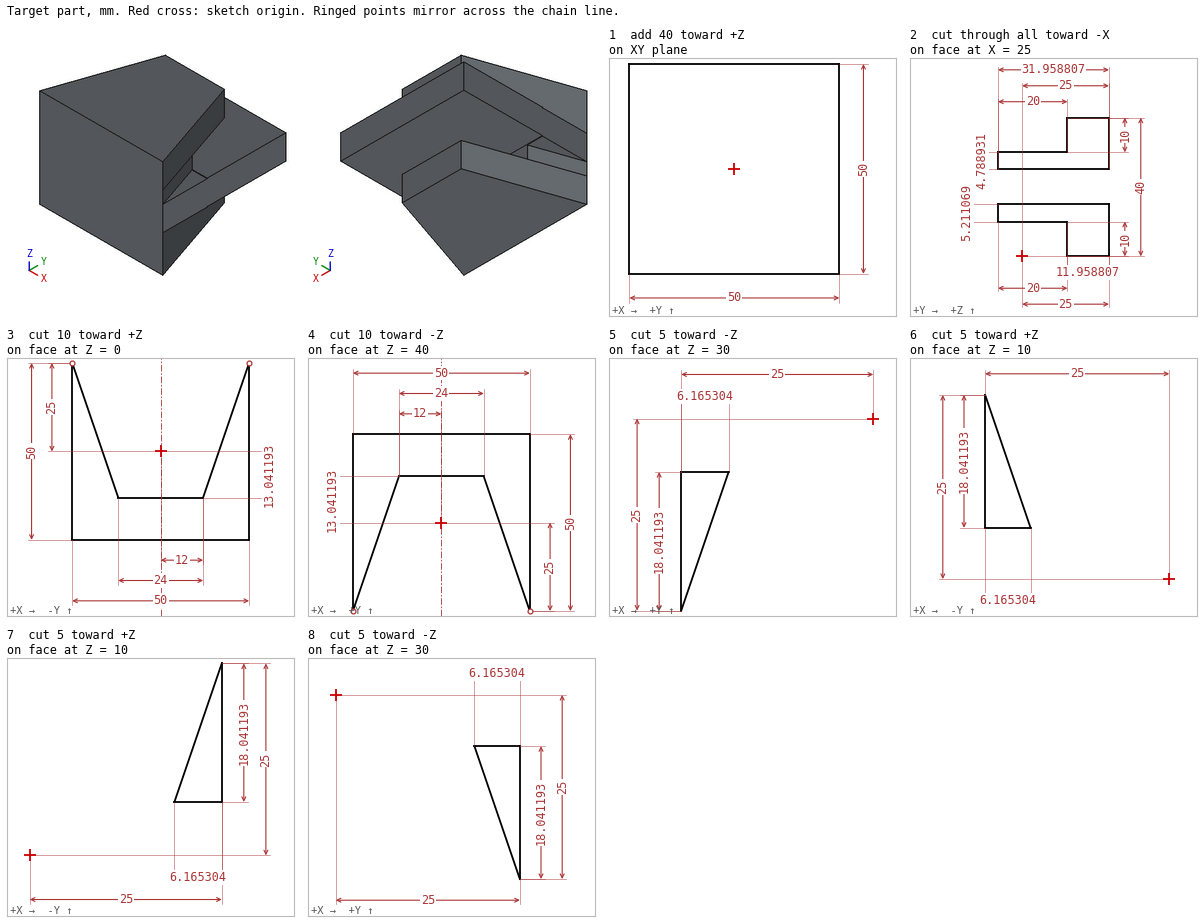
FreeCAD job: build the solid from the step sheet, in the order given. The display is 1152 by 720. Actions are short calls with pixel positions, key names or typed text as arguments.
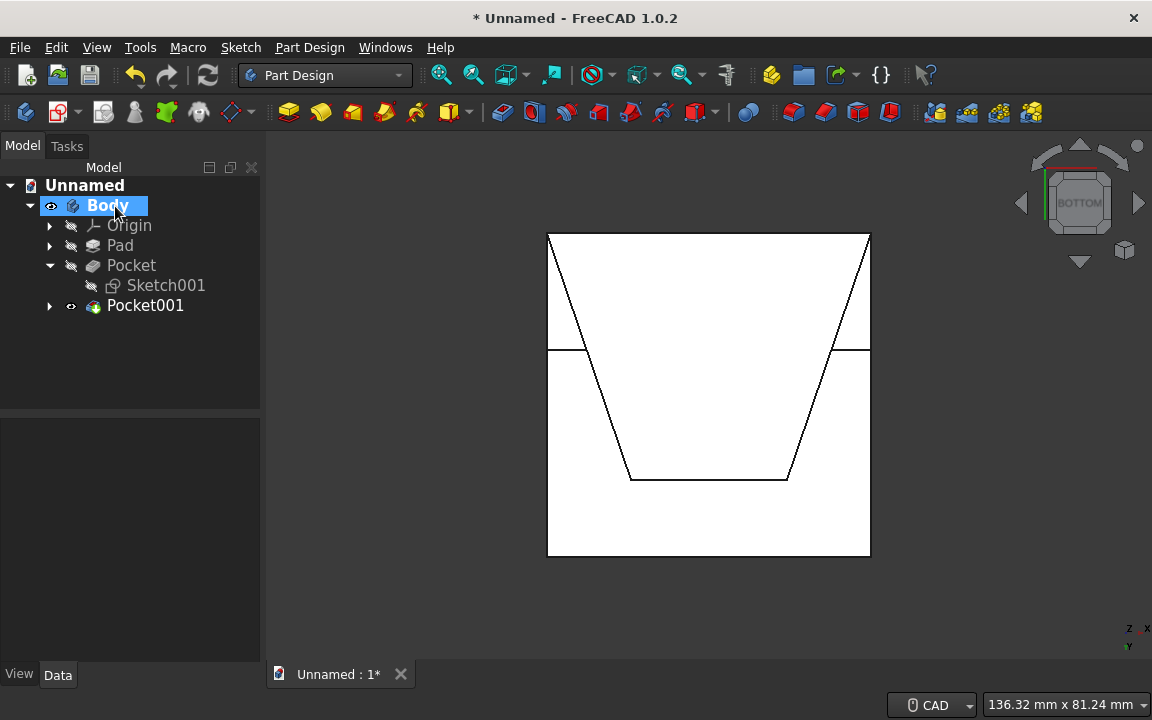
key(0)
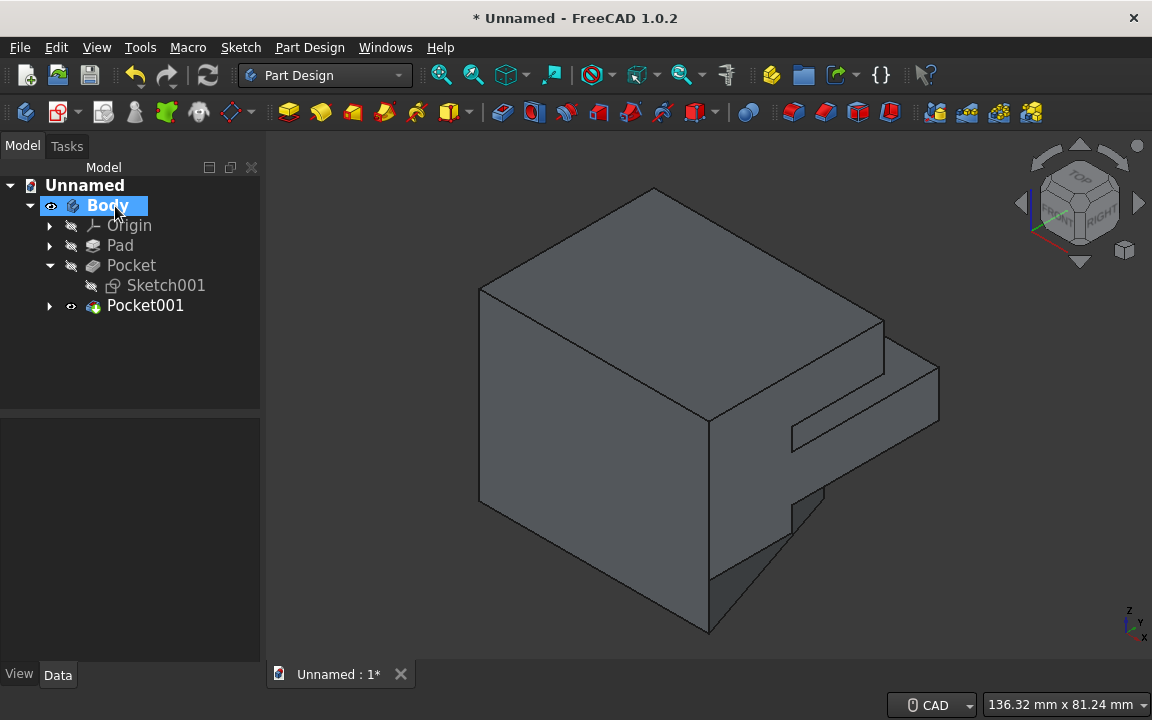
click(682, 304)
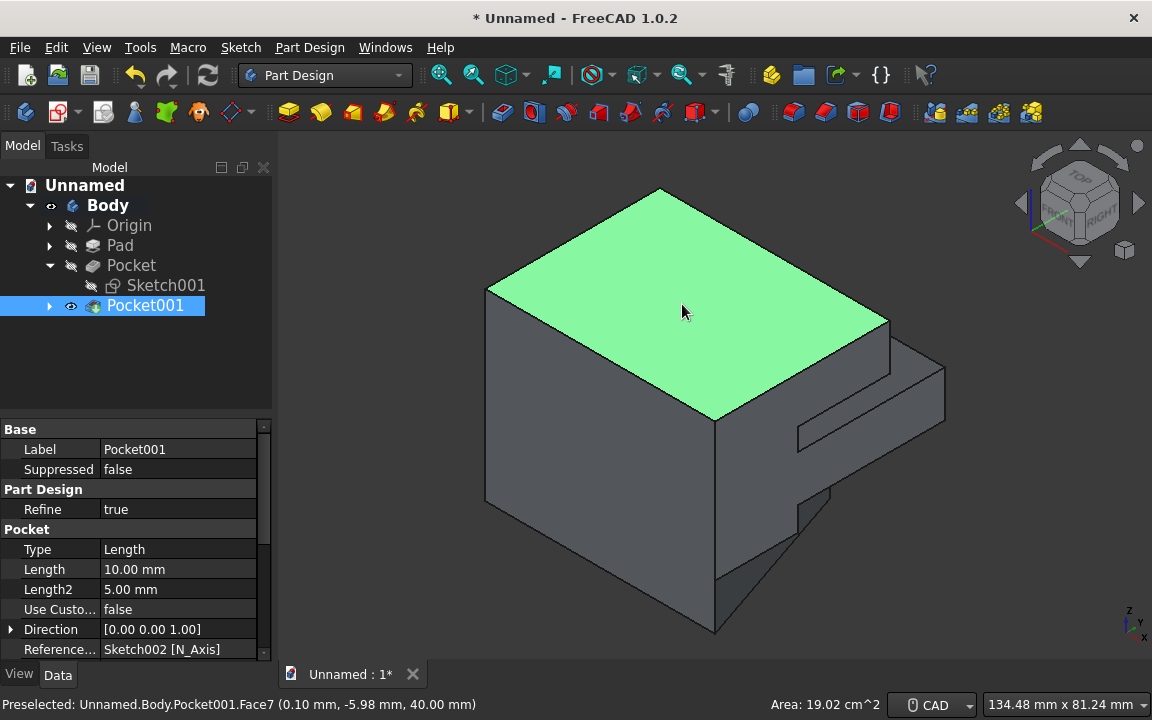
click(58, 112)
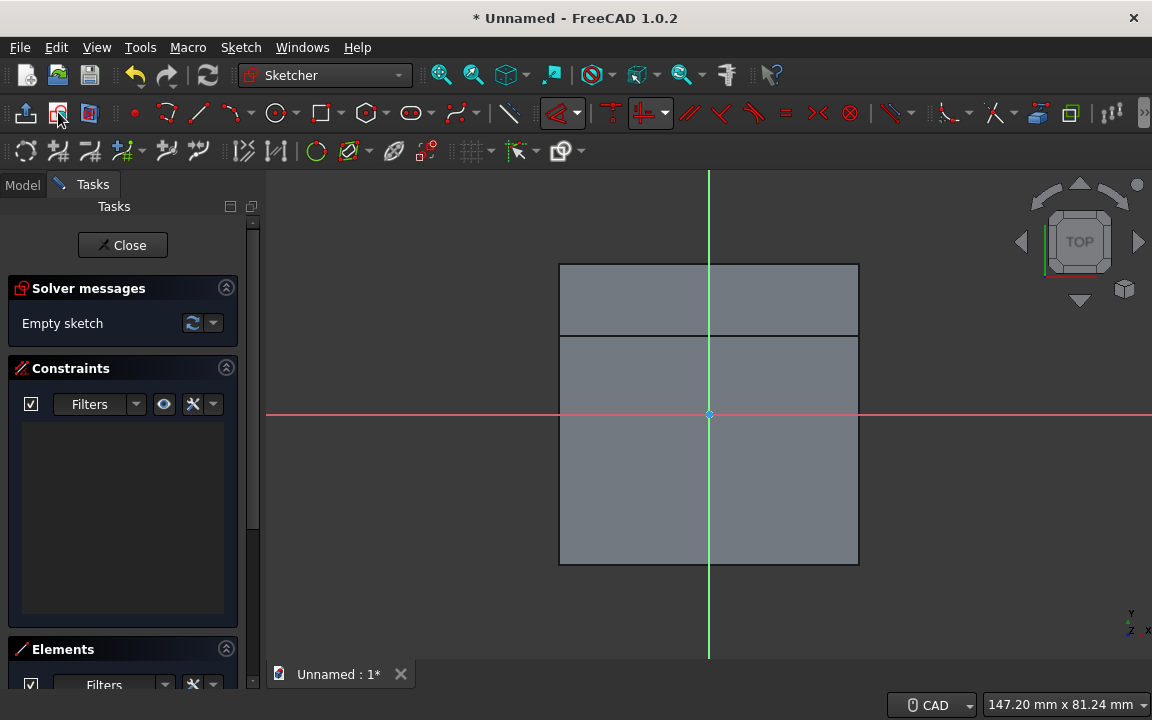
key(g)
key(m)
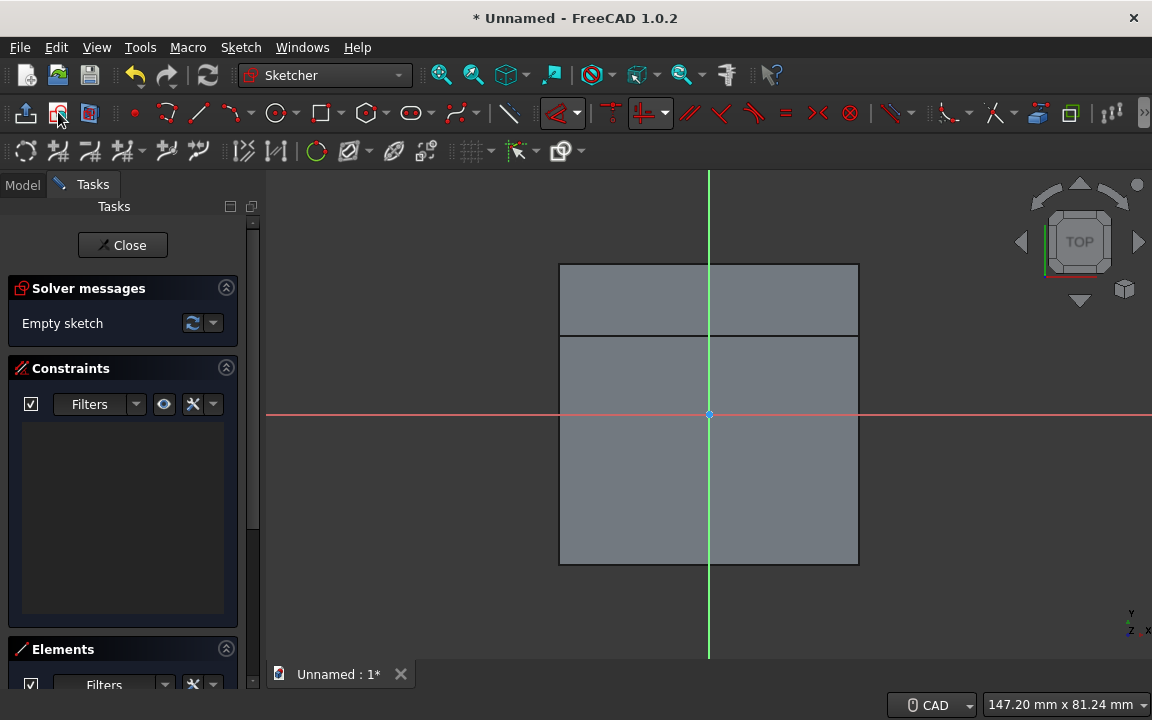
click(637, 336)
click(781, 336)
click(859, 565)
click(859, 264)
click(559, 264)
click(559, 565)
click(637, 337)
key(Escape)
key(Escape)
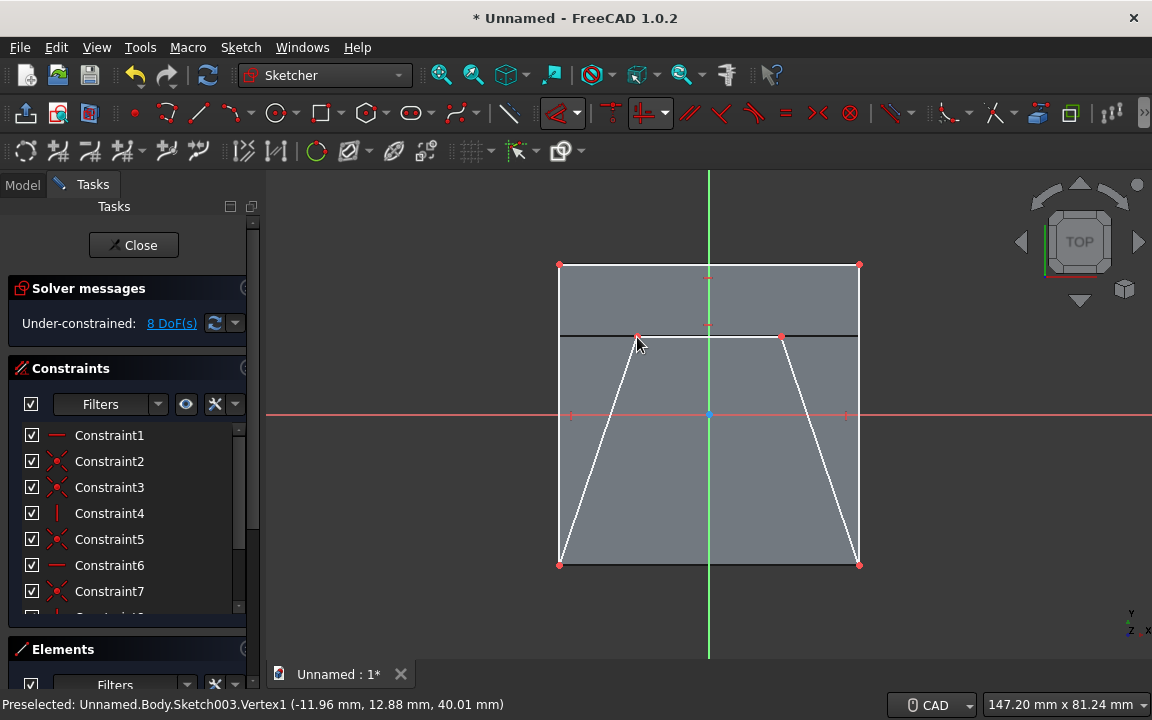
click(859, 566)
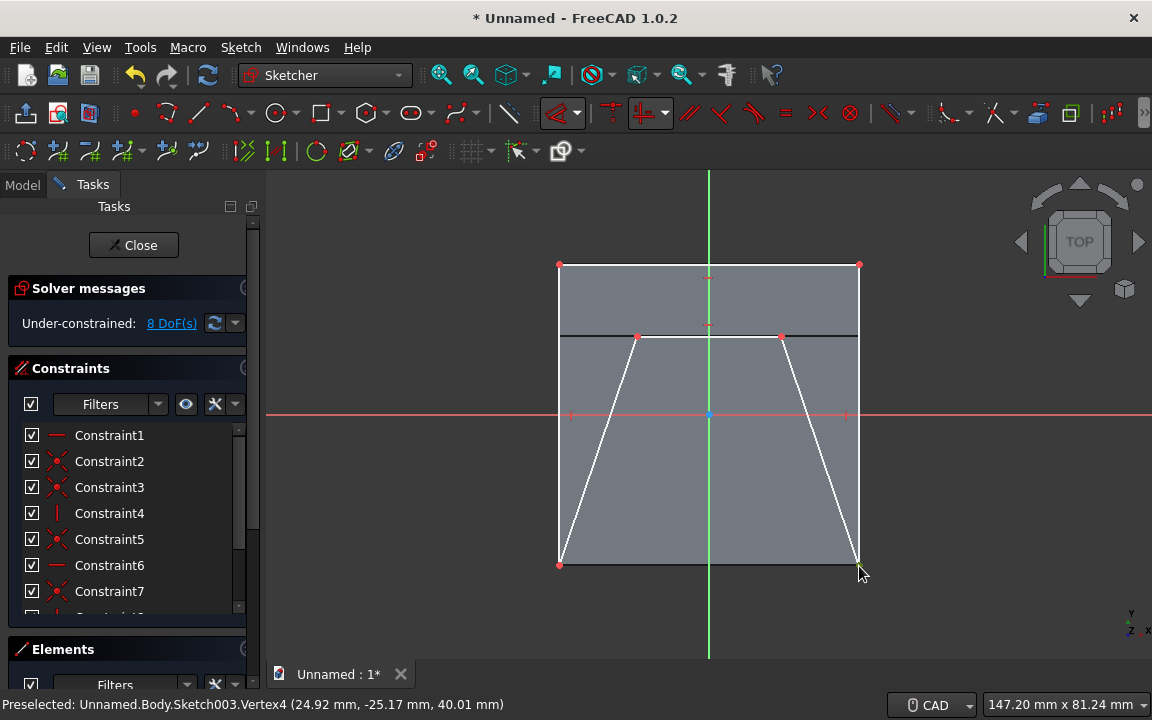
click(559, 566)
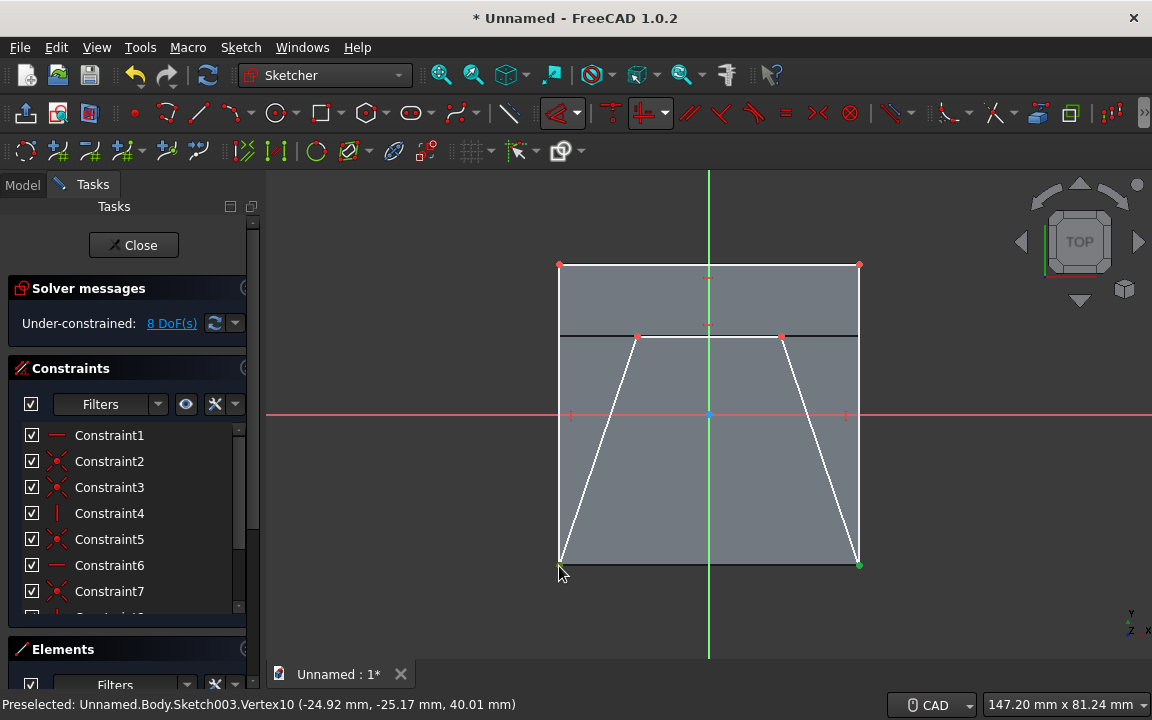
click(709, 600)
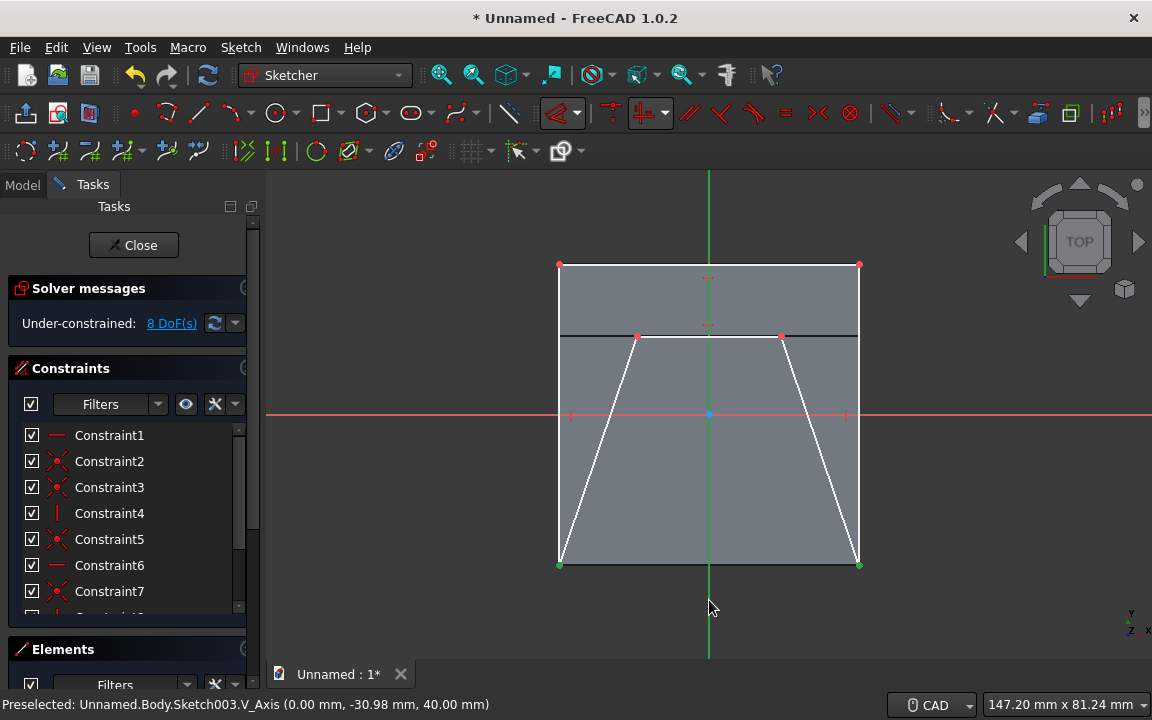
key(s)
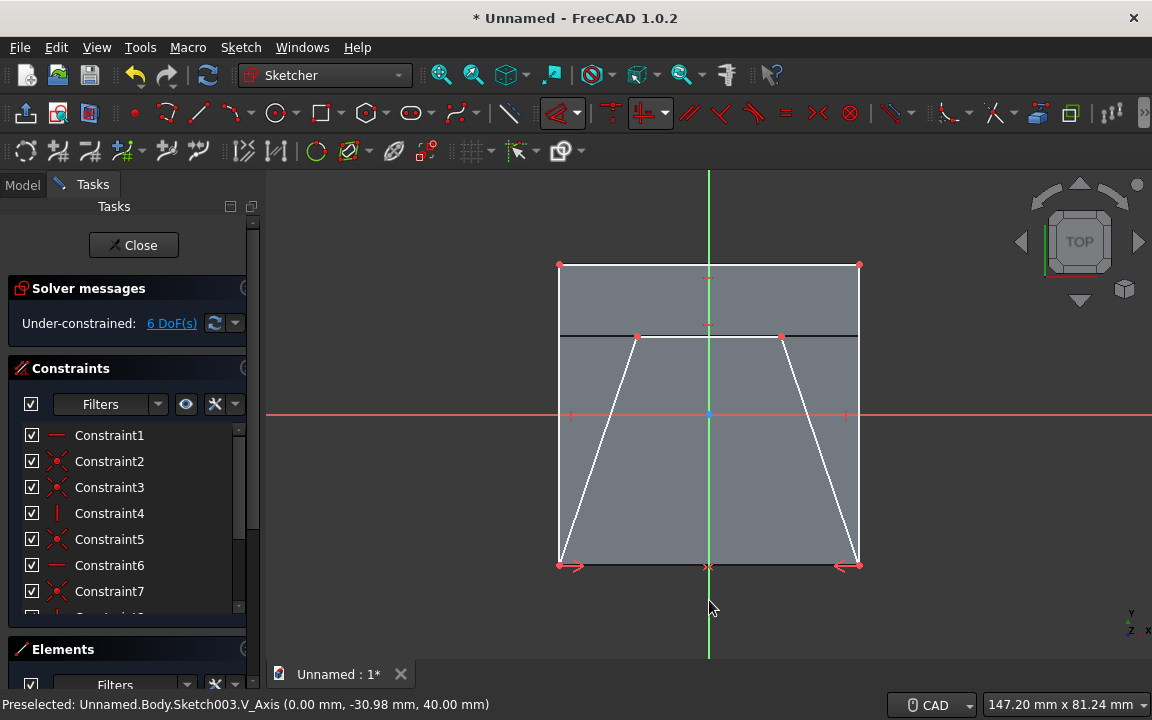
click(680, 337)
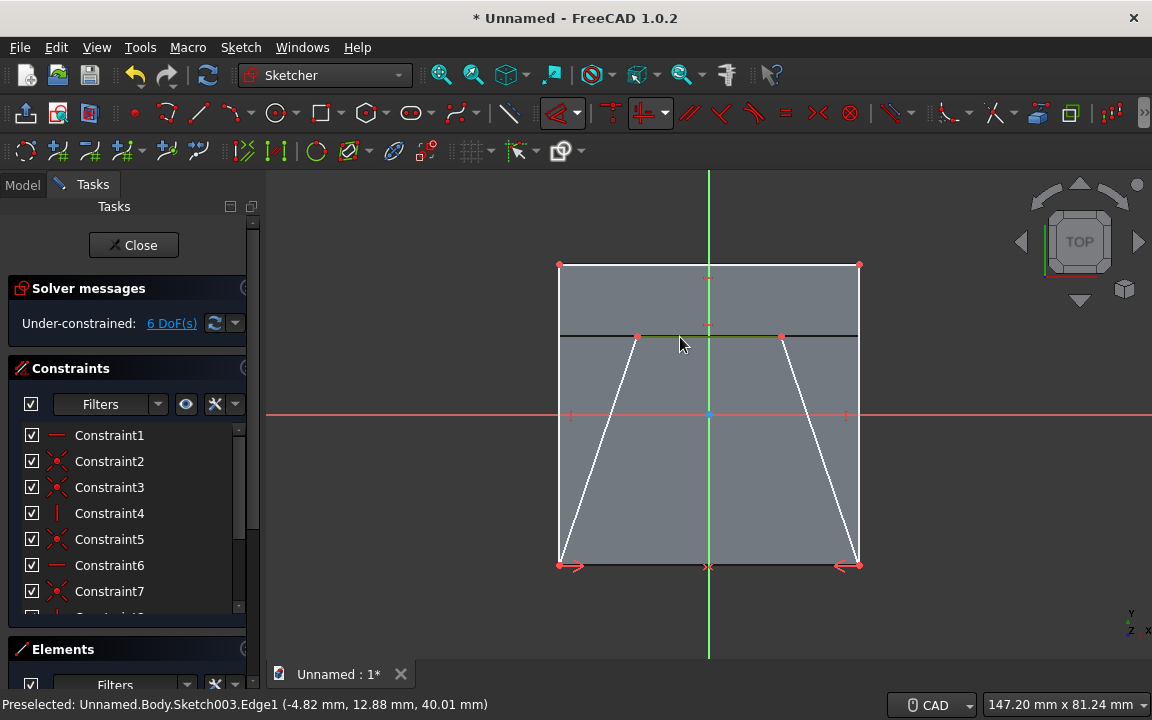
key(l)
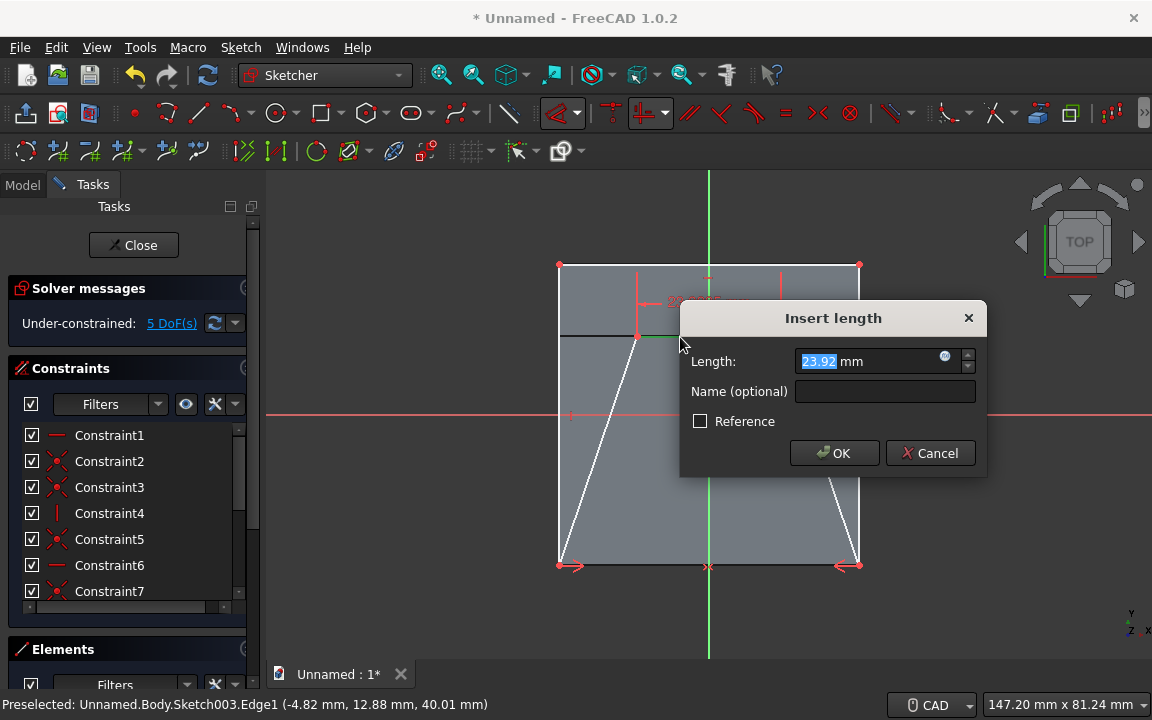
text(24)
key(Return)